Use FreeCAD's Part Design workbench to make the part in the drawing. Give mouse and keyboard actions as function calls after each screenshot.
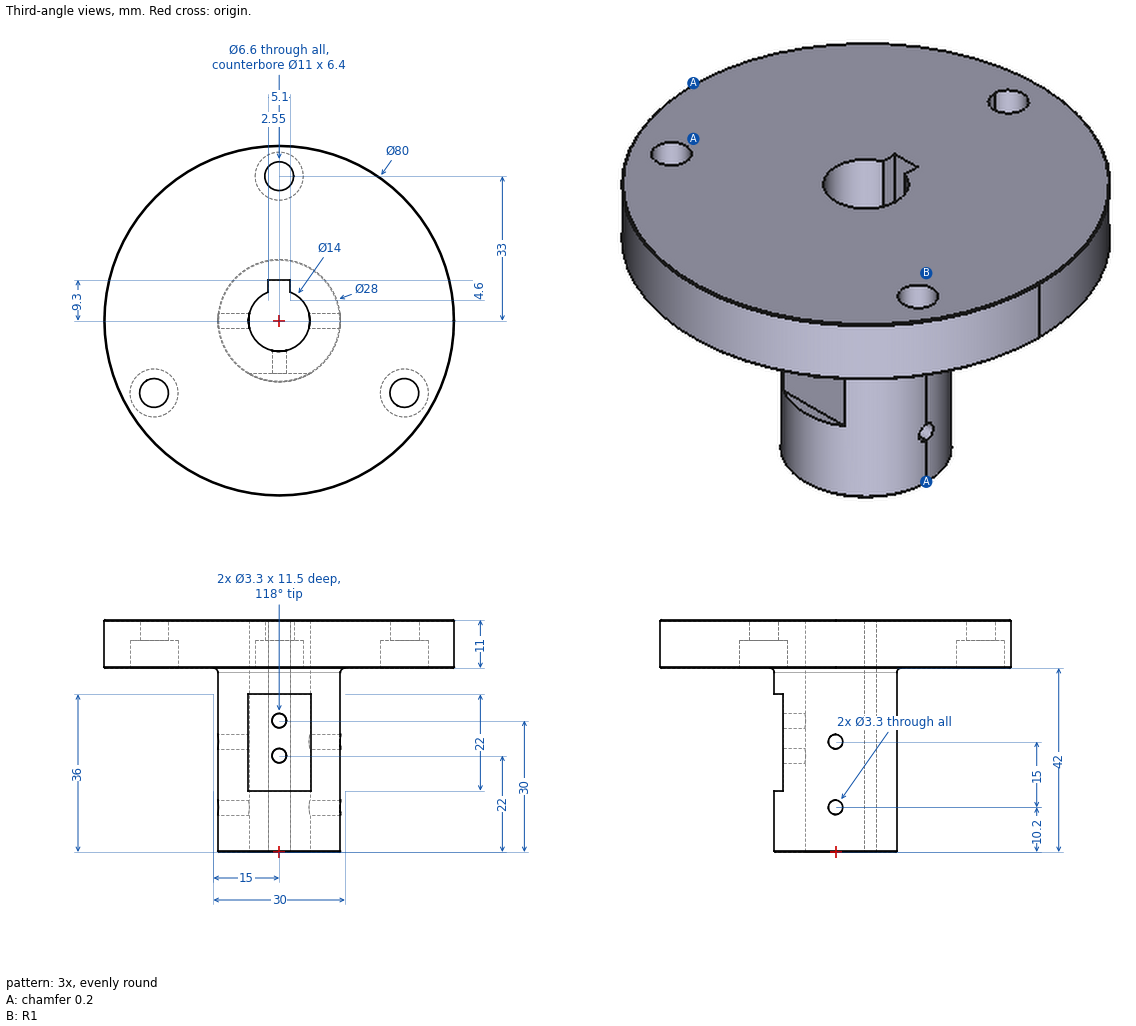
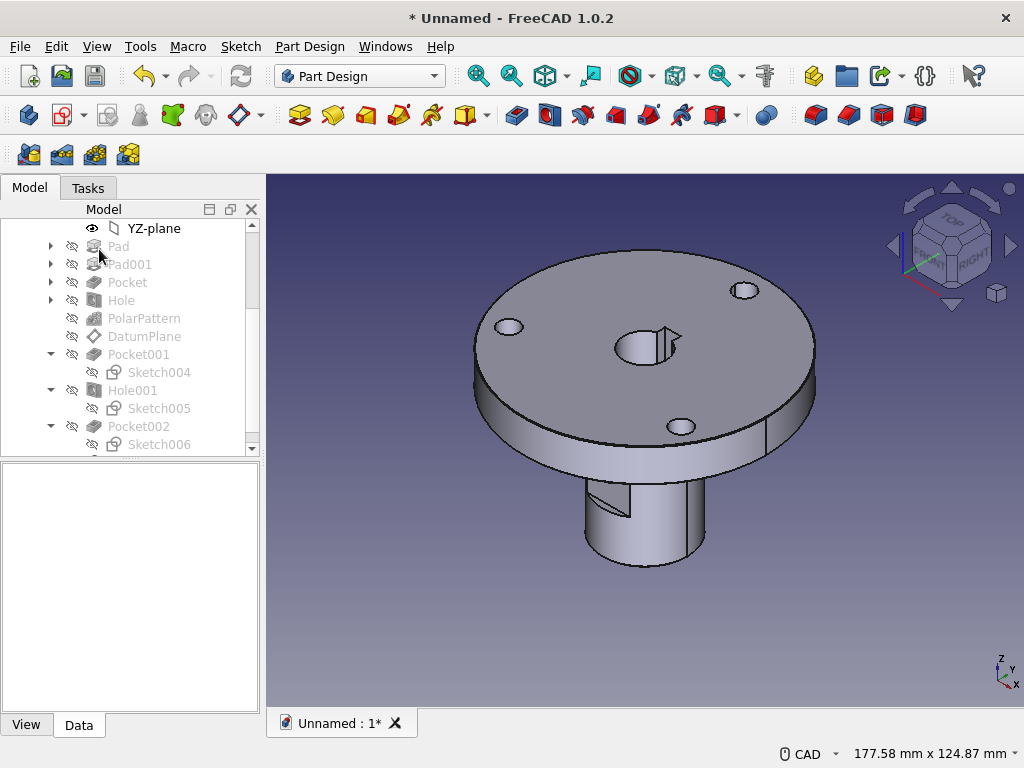
key(2)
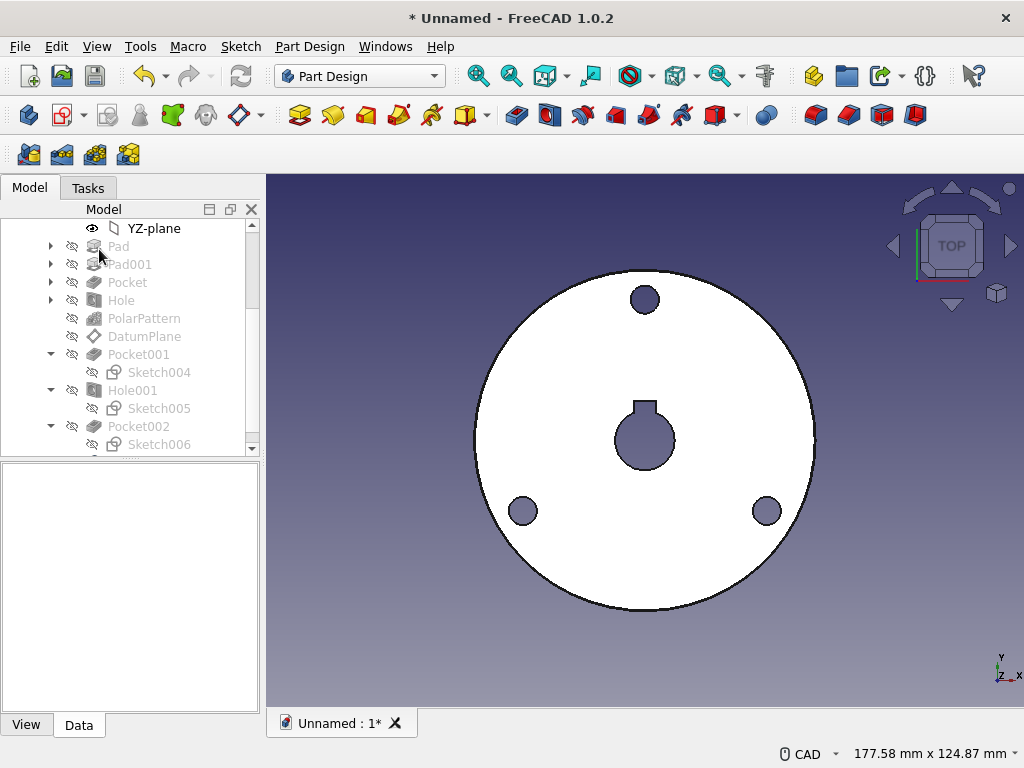
key(1)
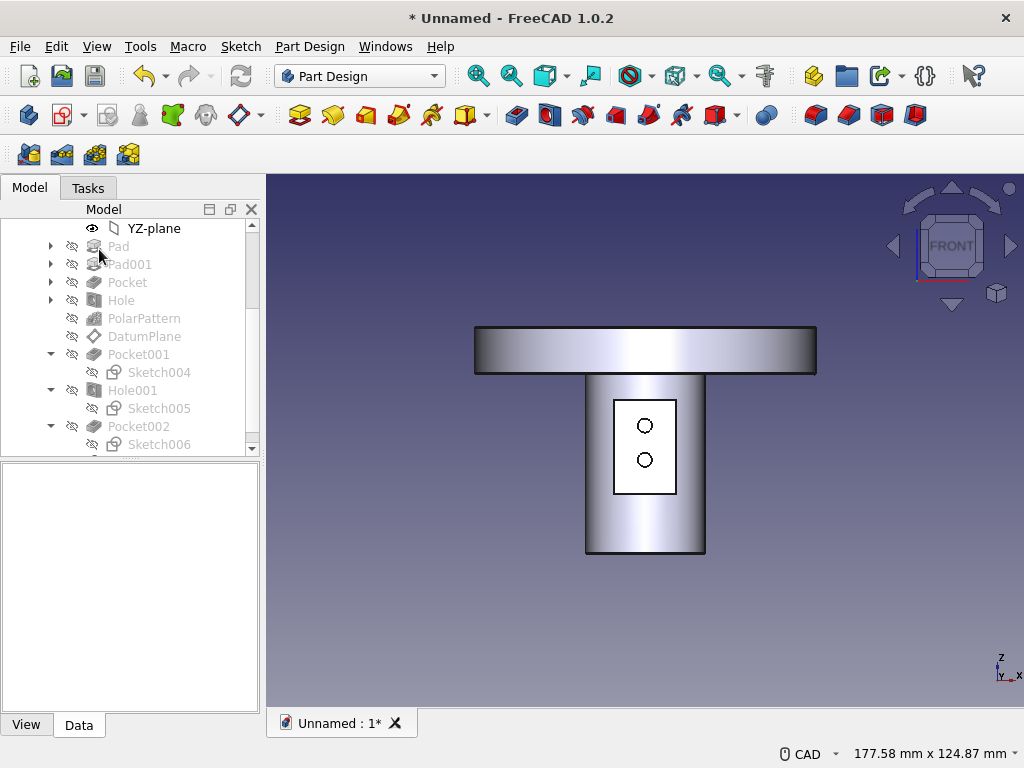
key(3)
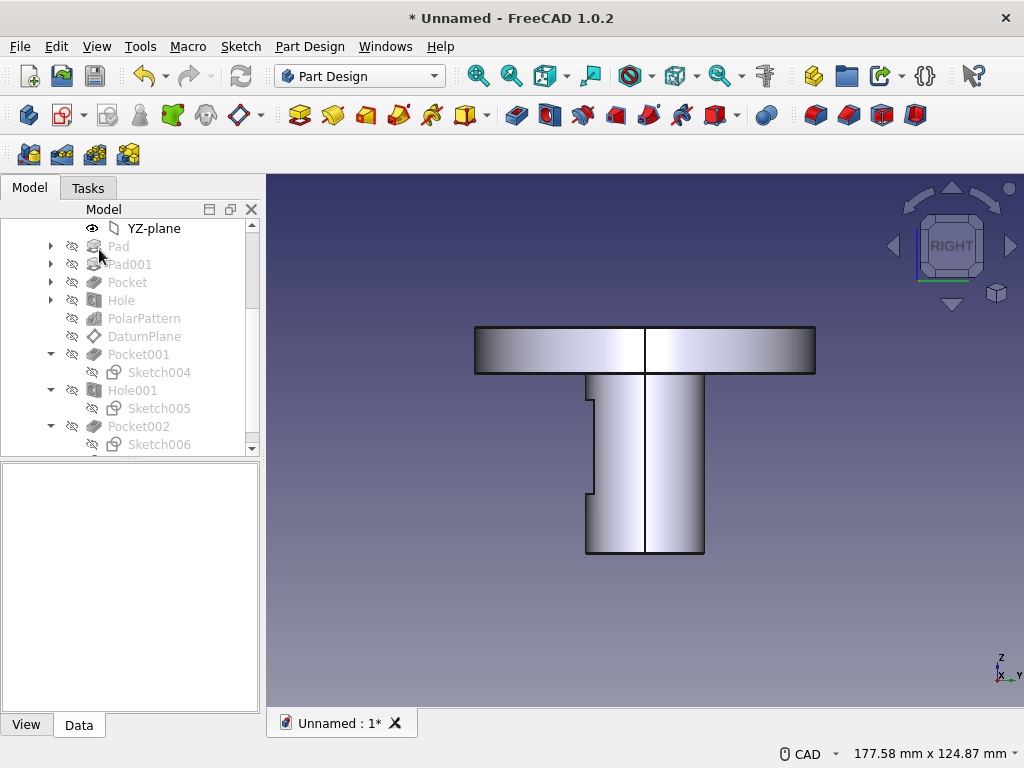
key(5)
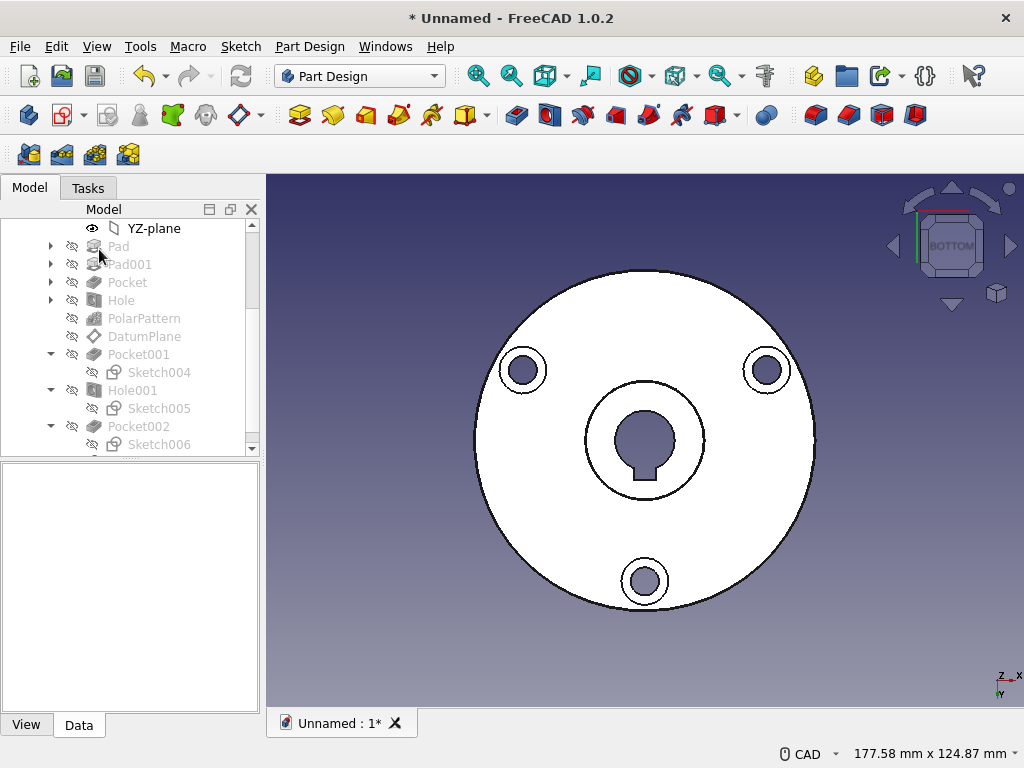
key(4)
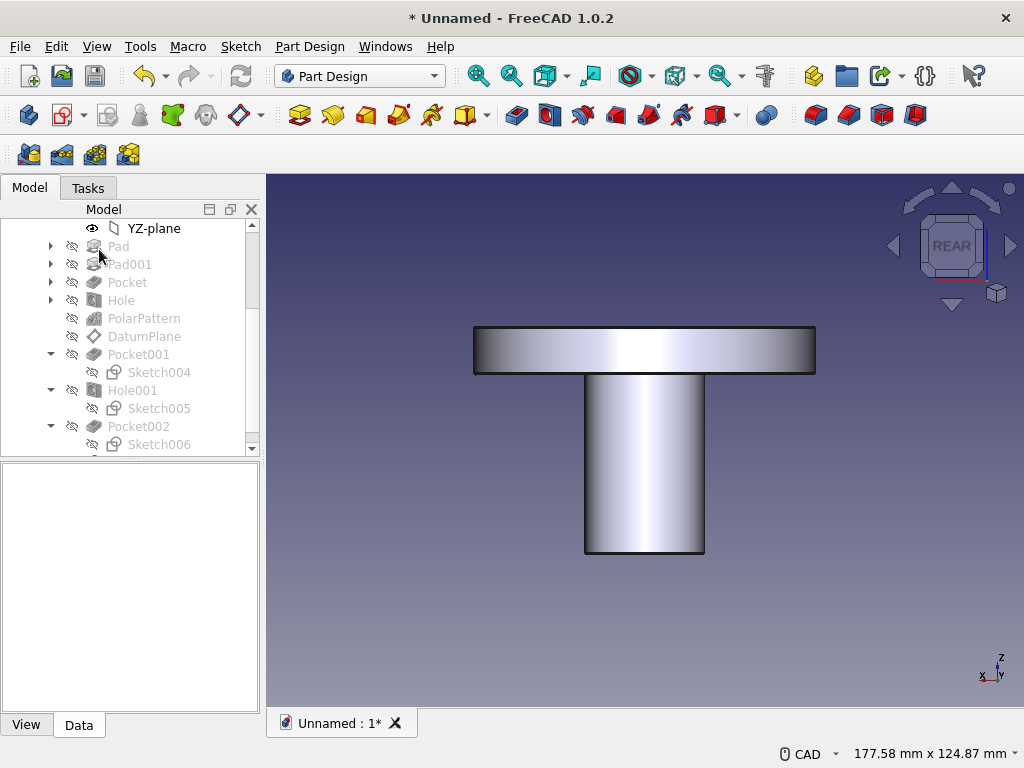
key(6)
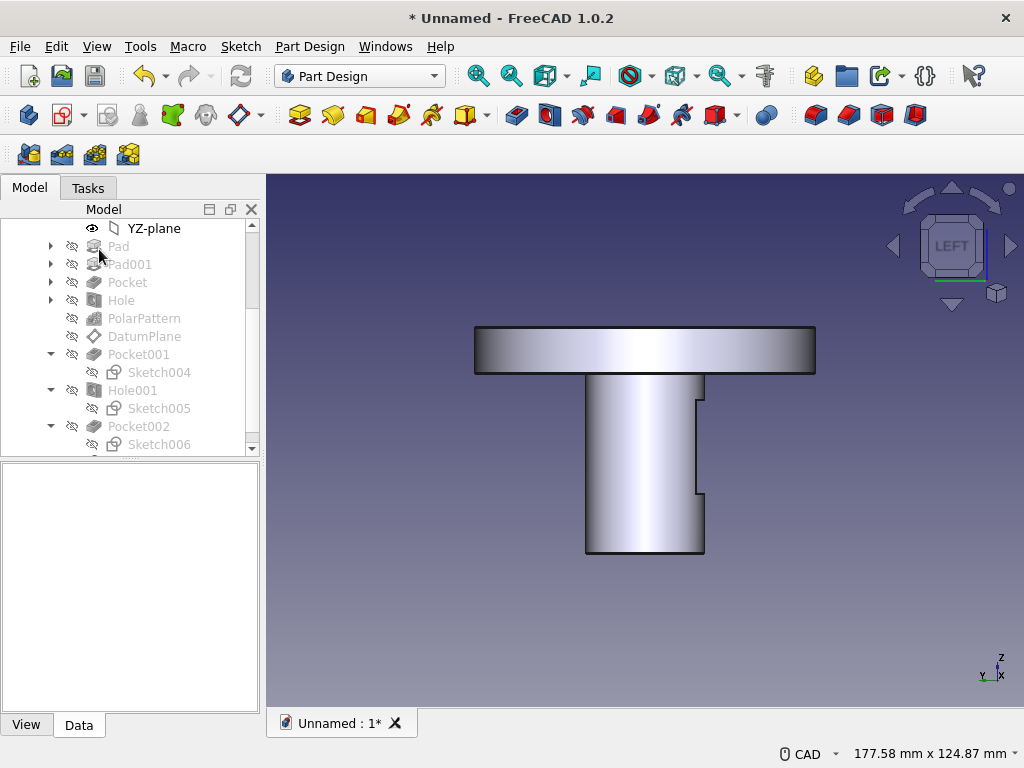
key(v)
key(3)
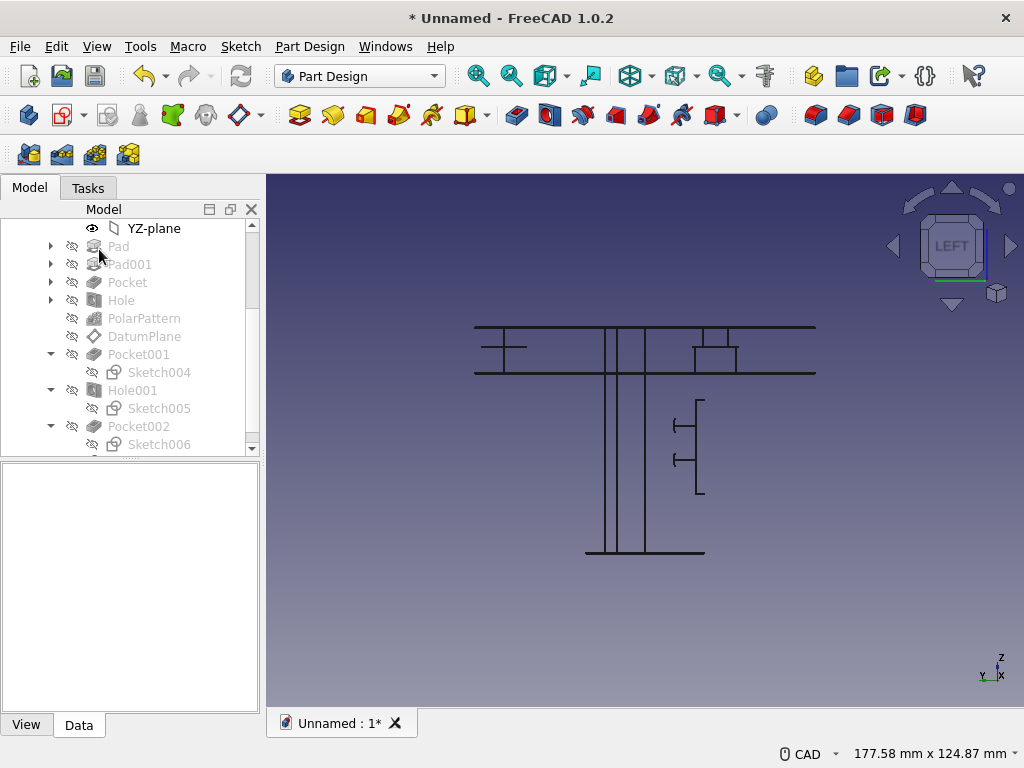
key(0)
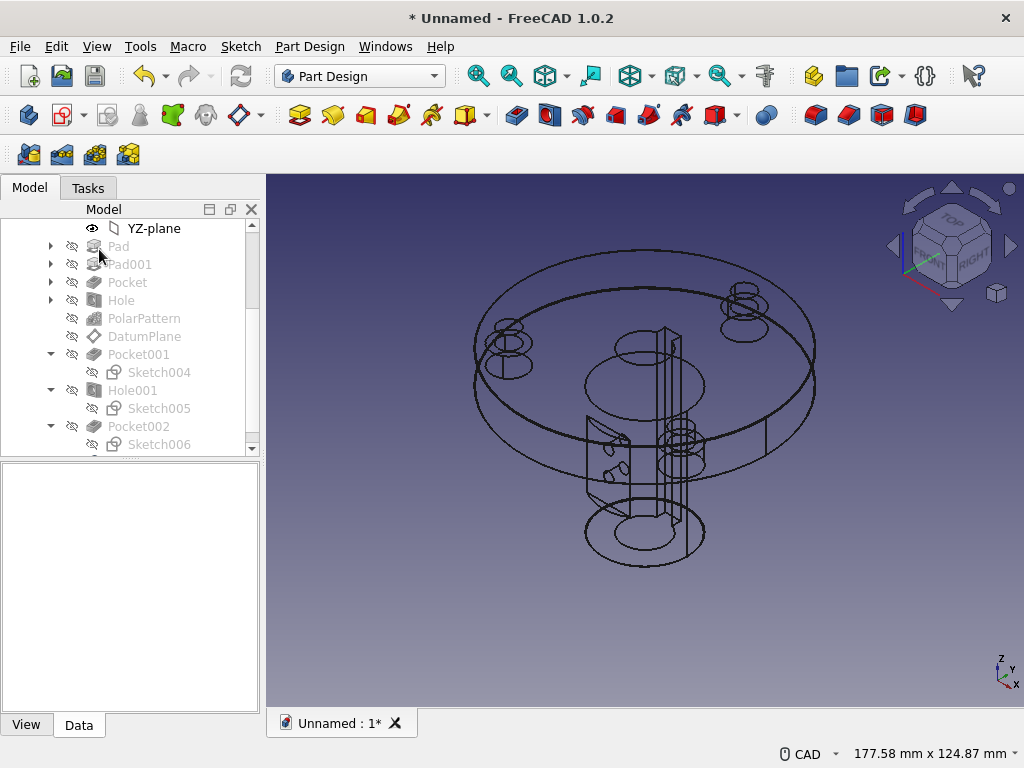
click(603, 361)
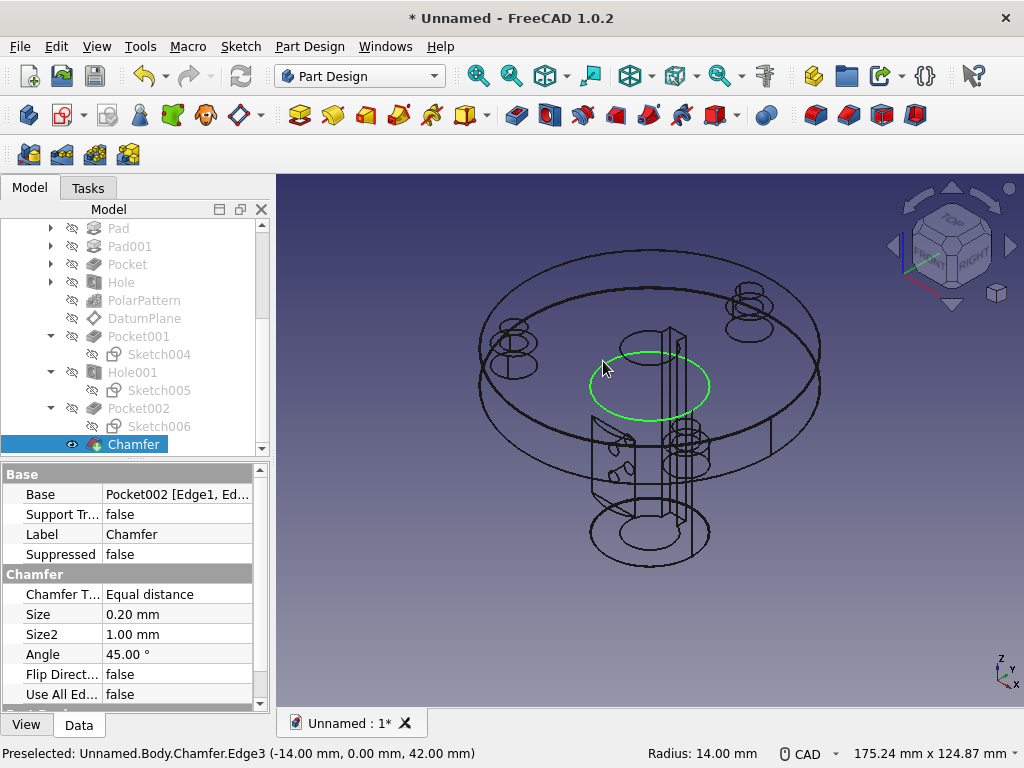
key(v)
key(1)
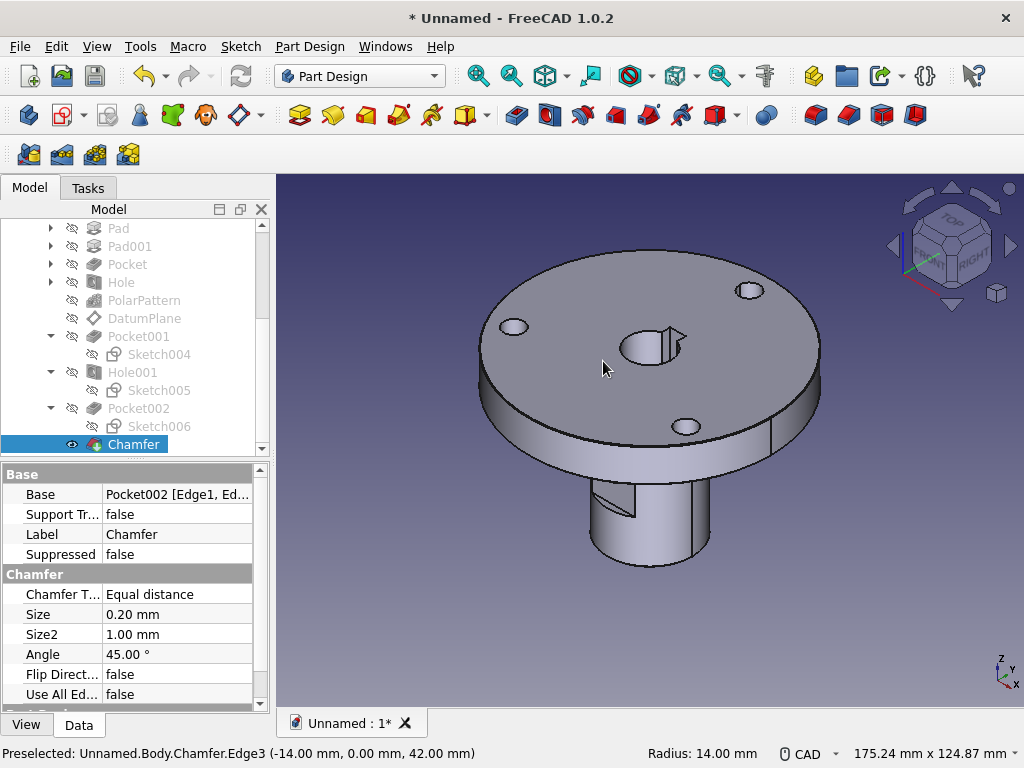
click(816, 116)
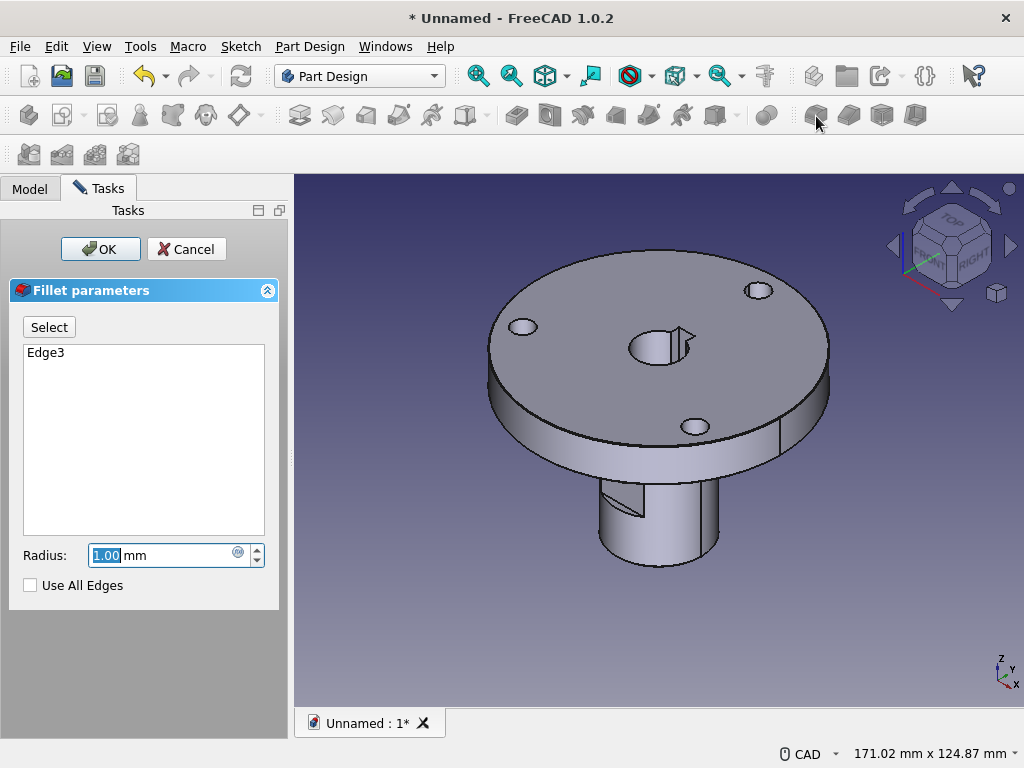
text(1)
key(Tab)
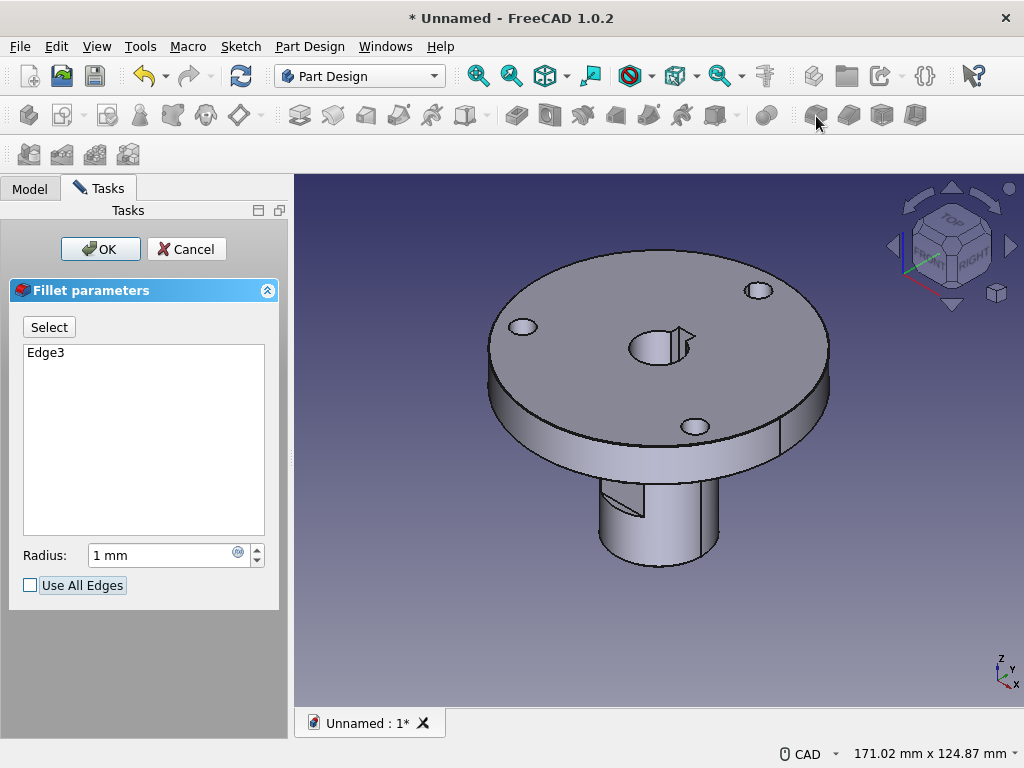
click(101, 249)